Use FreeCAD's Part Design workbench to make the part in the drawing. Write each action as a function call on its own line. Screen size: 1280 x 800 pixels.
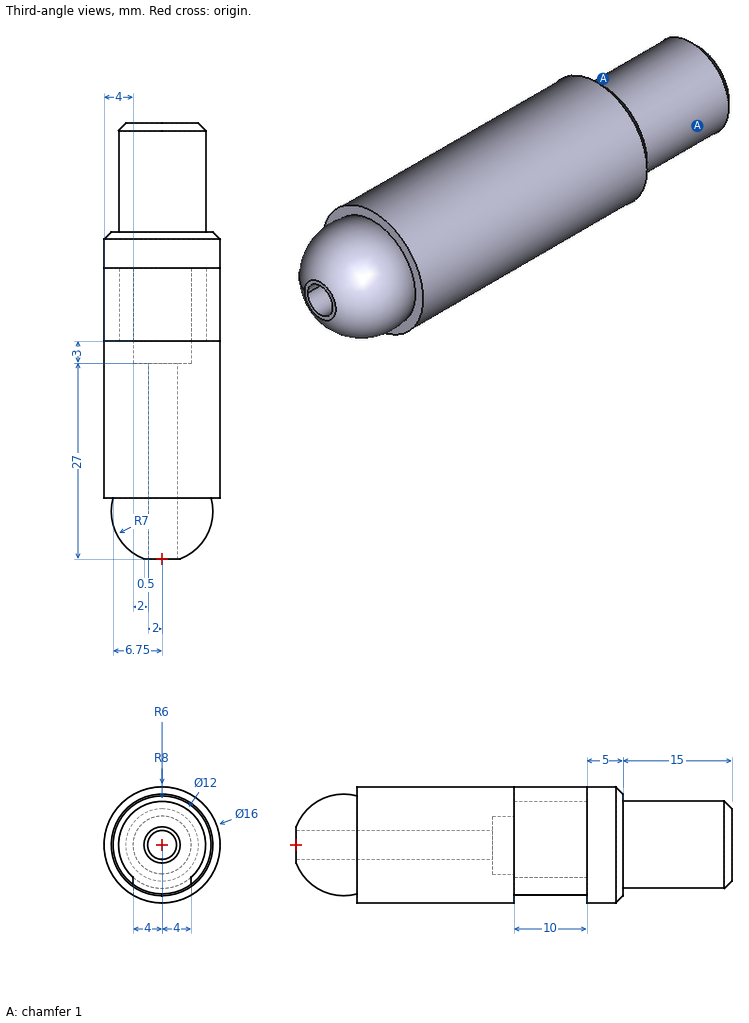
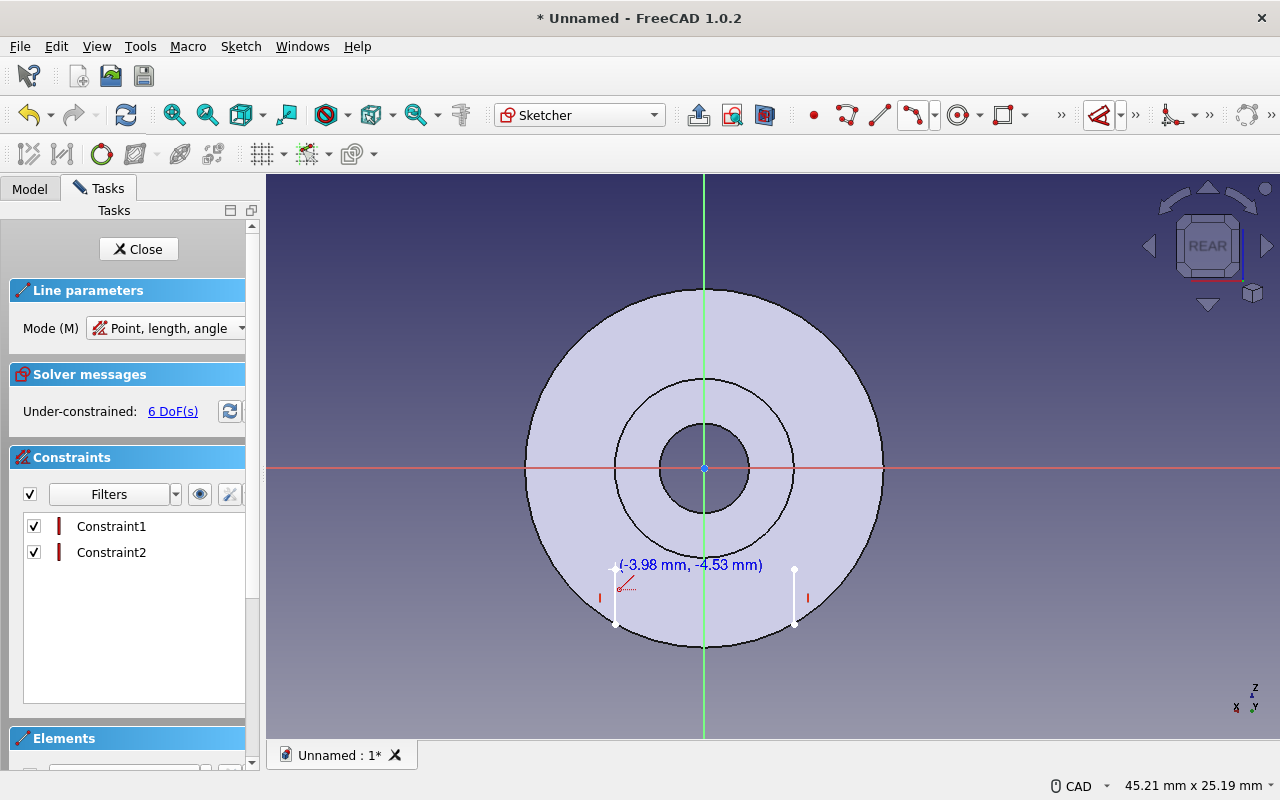
click(912, 116)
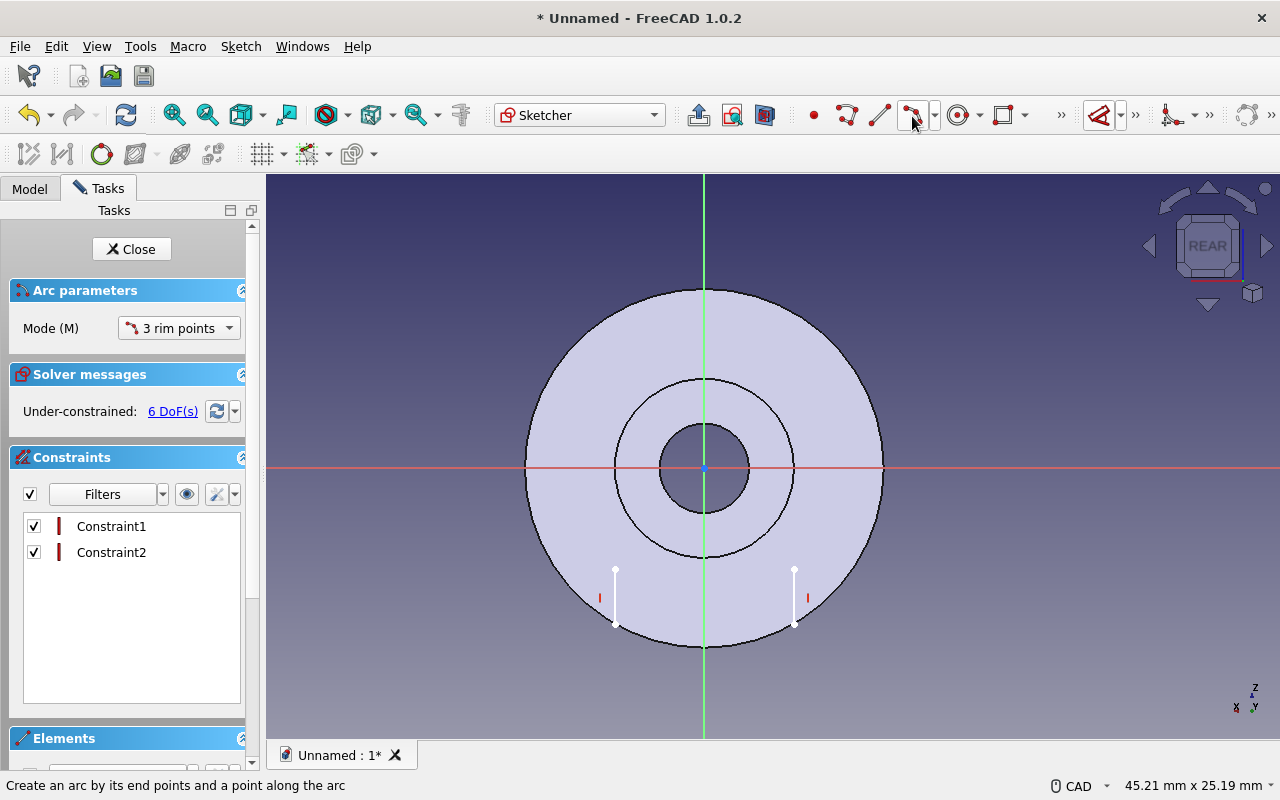
click(794, 625)
click(615, 625)
click(794, 313)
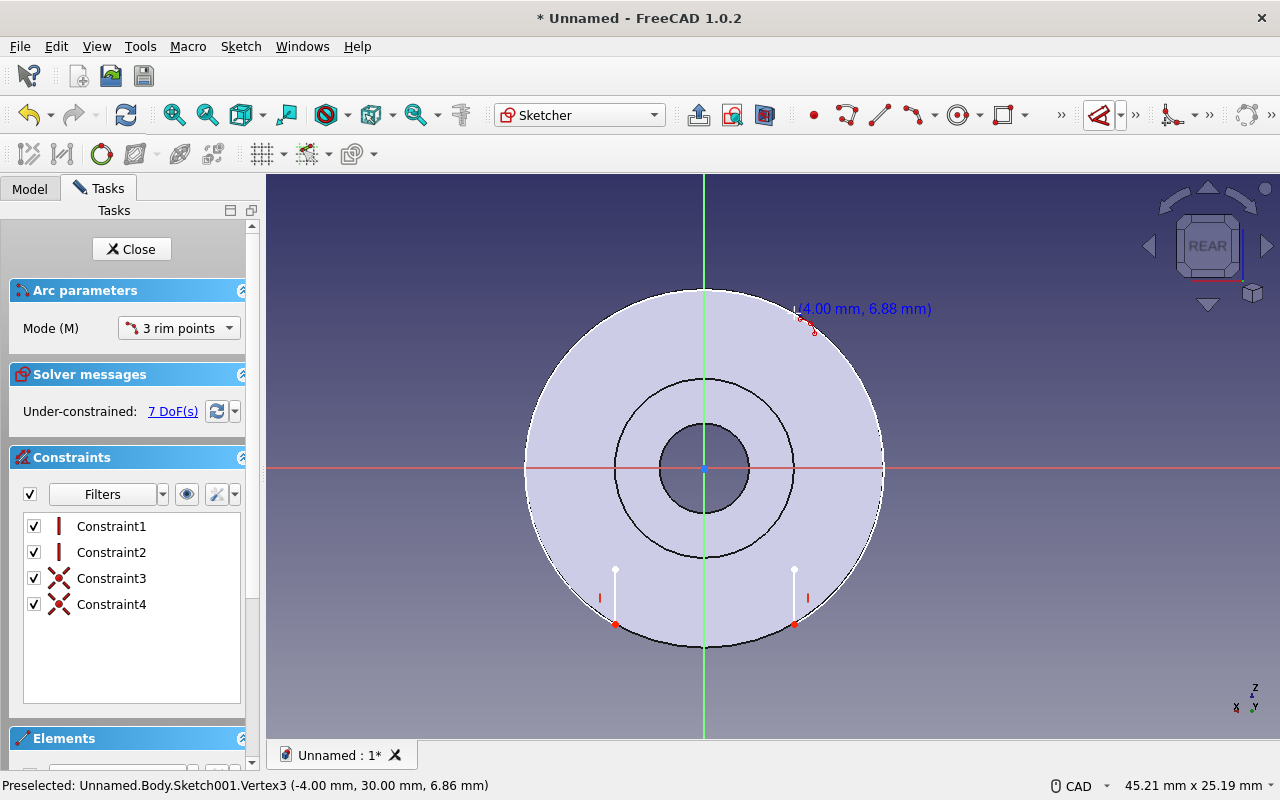
click(615, 570)
click(794, 570)
click(767, 349)
key(Escape)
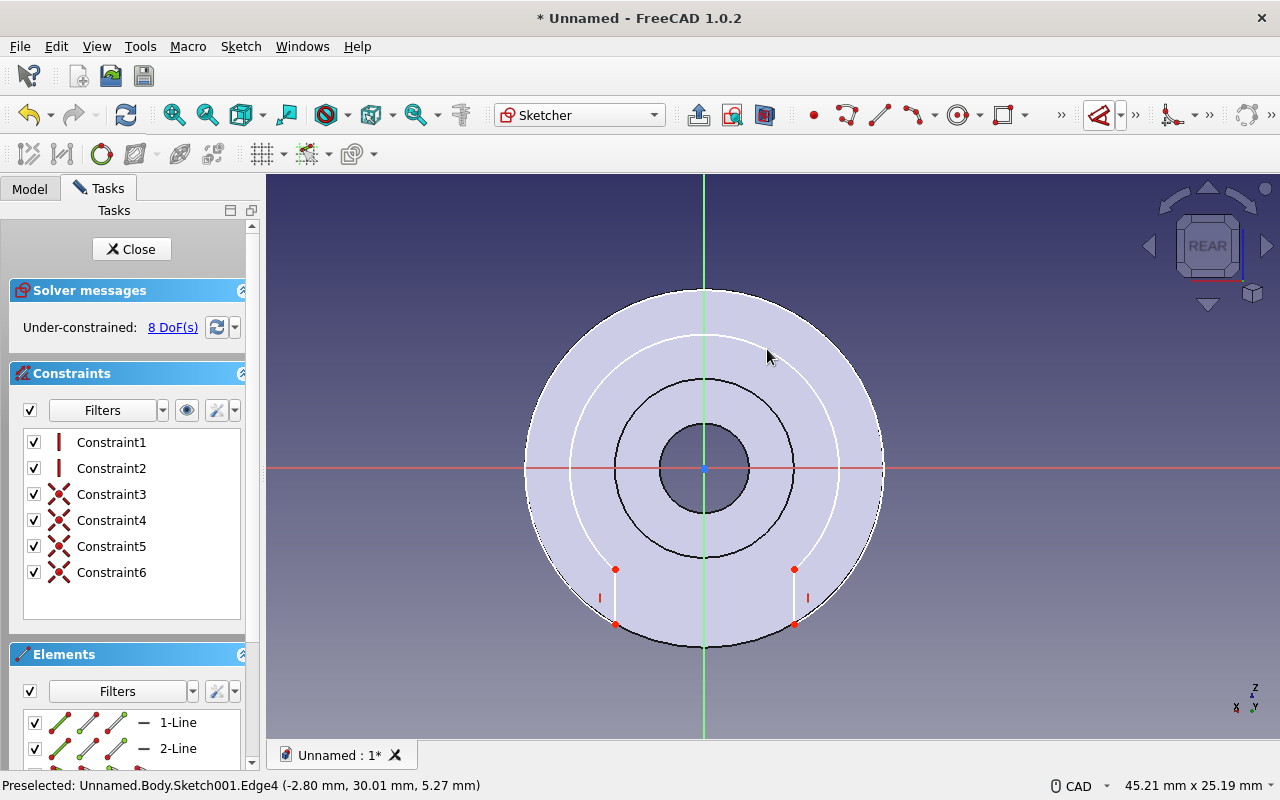
click(860, 380)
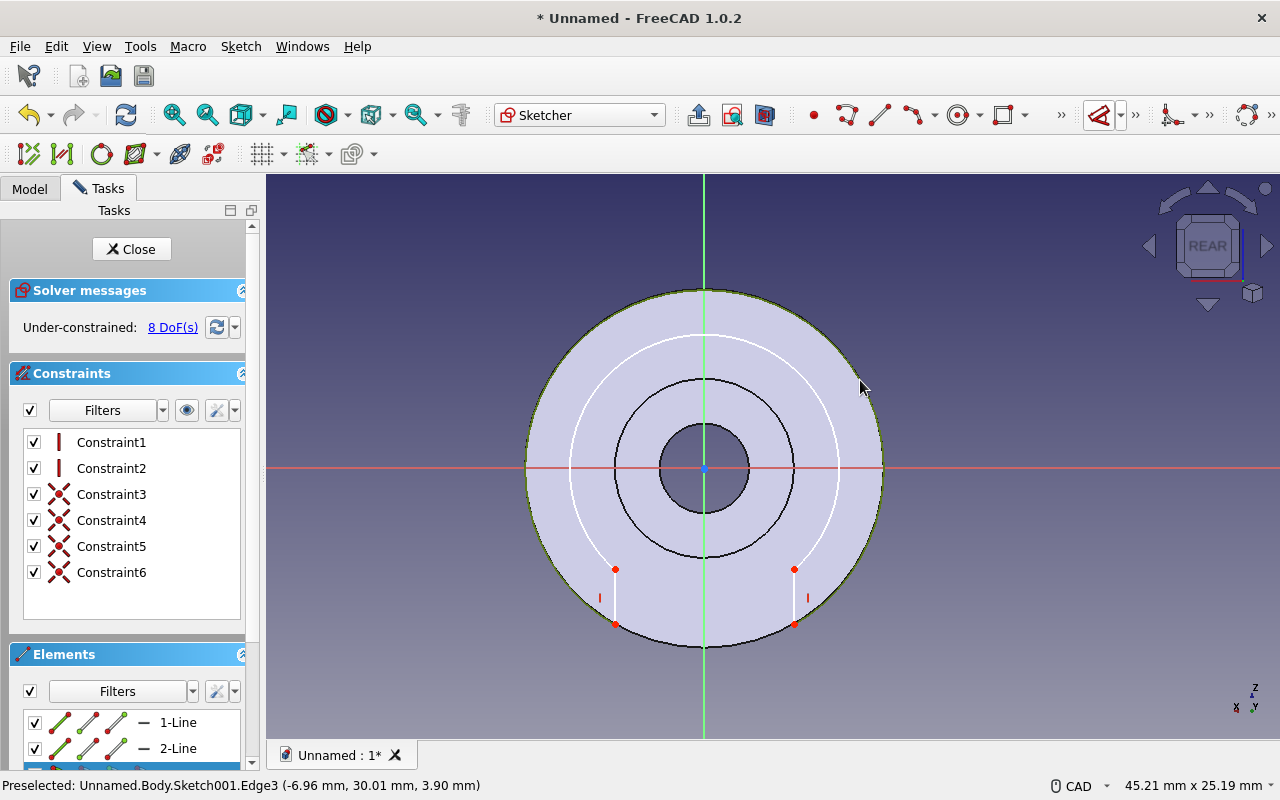
click(815, 393)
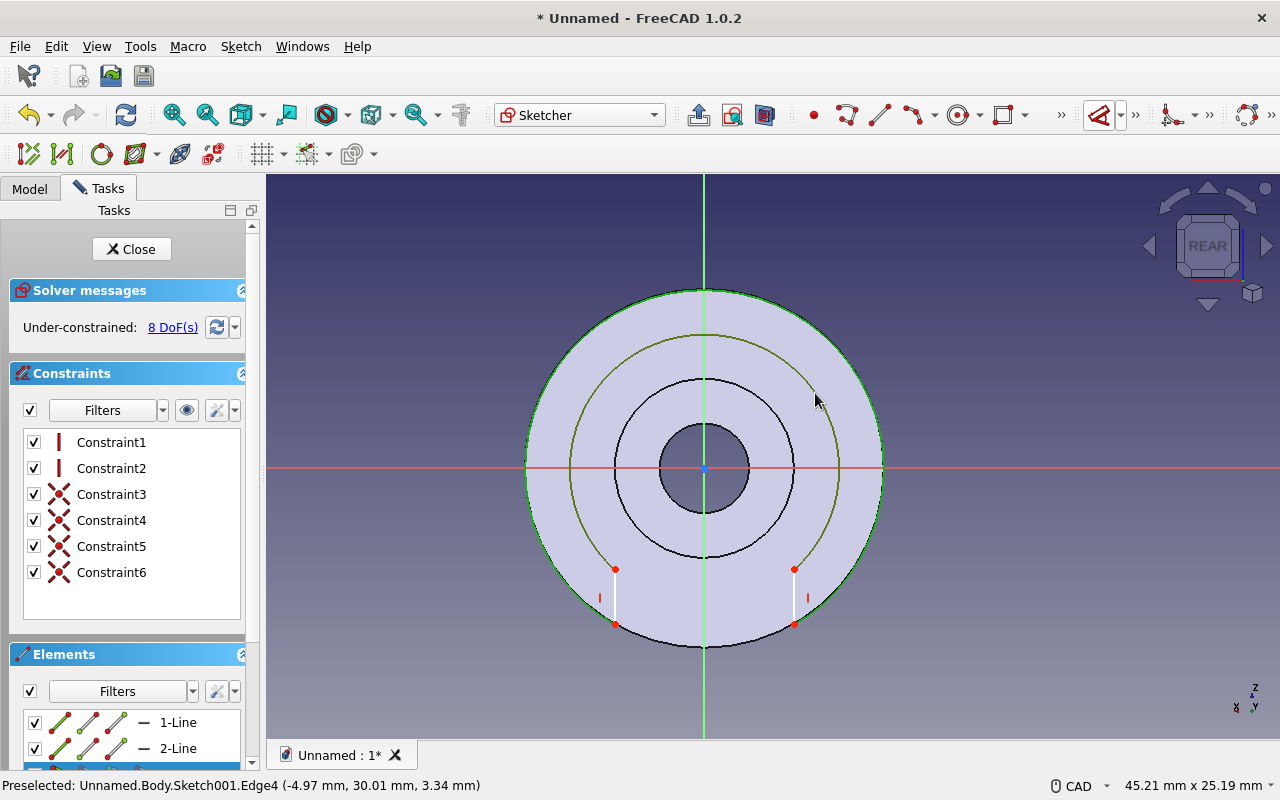
key(c)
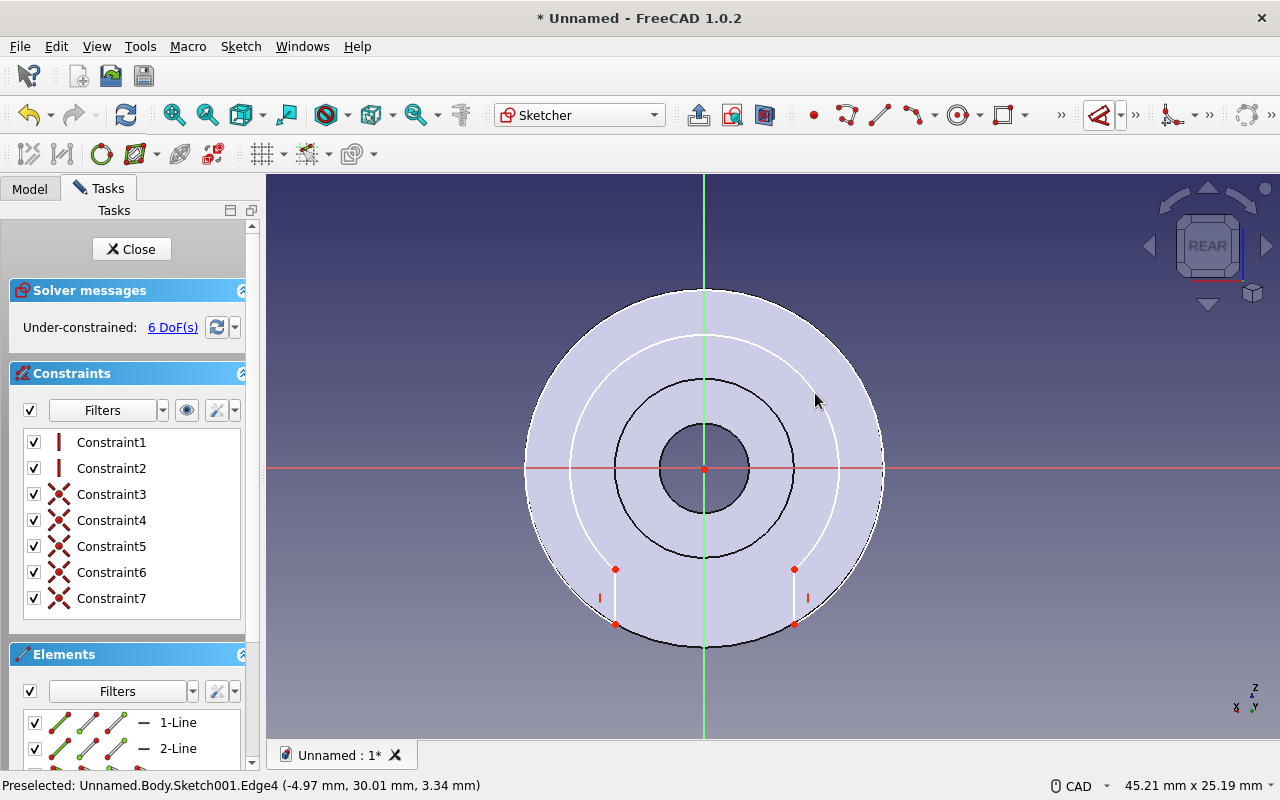
drag(694, 458, 714, 479)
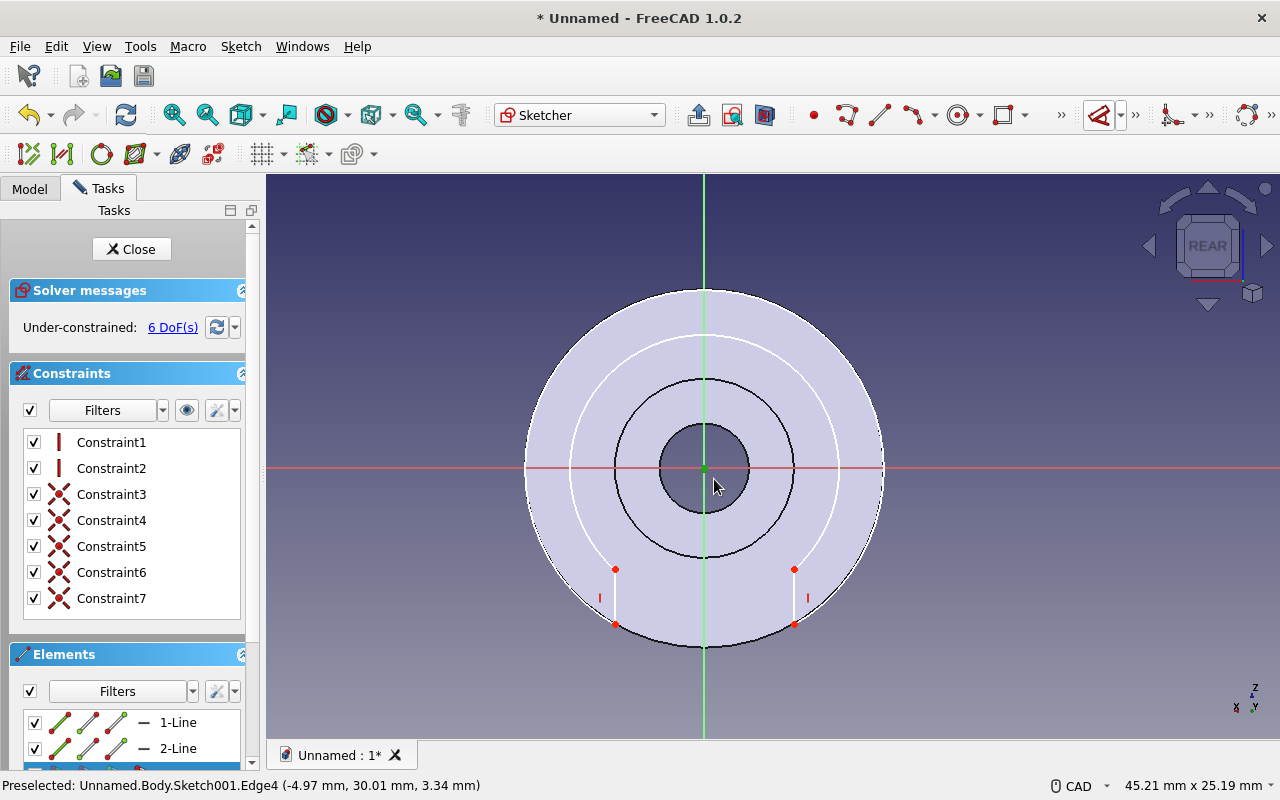
key(c)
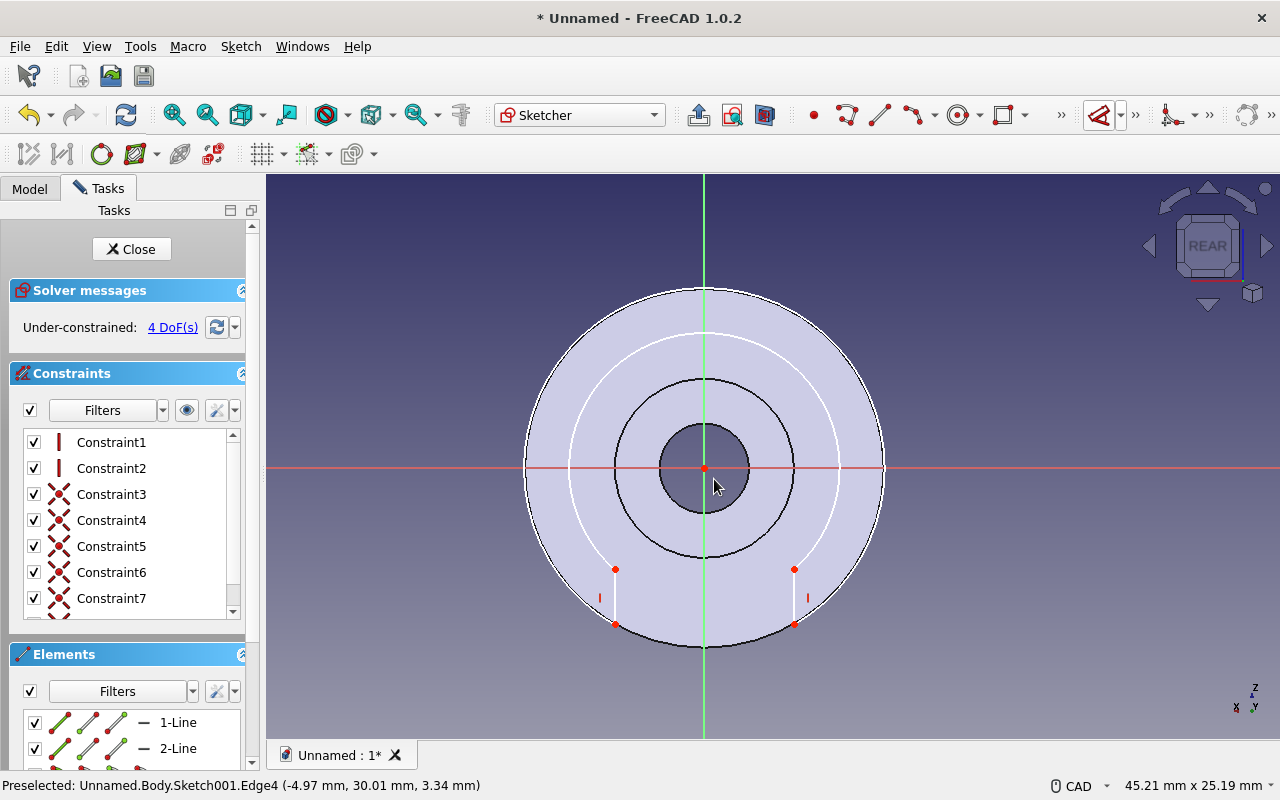
click(861, 378)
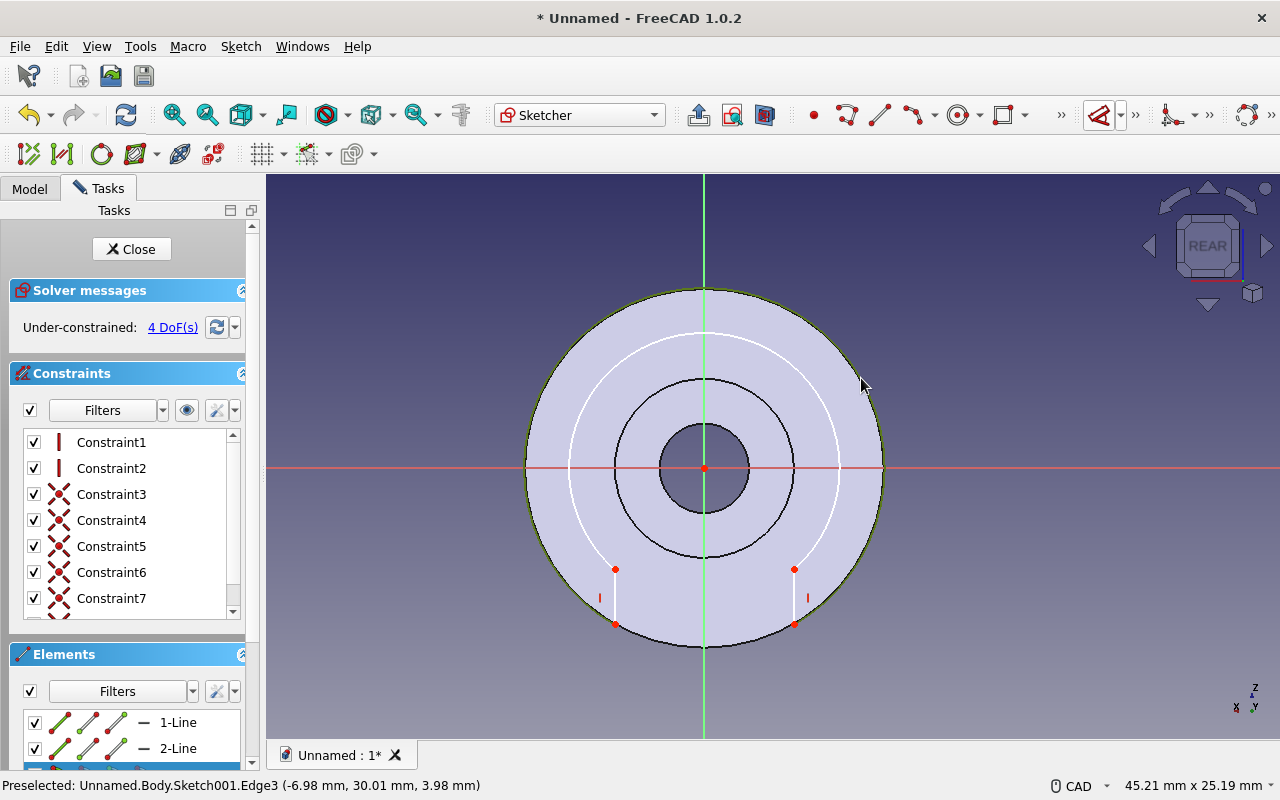
click(1120, 116)